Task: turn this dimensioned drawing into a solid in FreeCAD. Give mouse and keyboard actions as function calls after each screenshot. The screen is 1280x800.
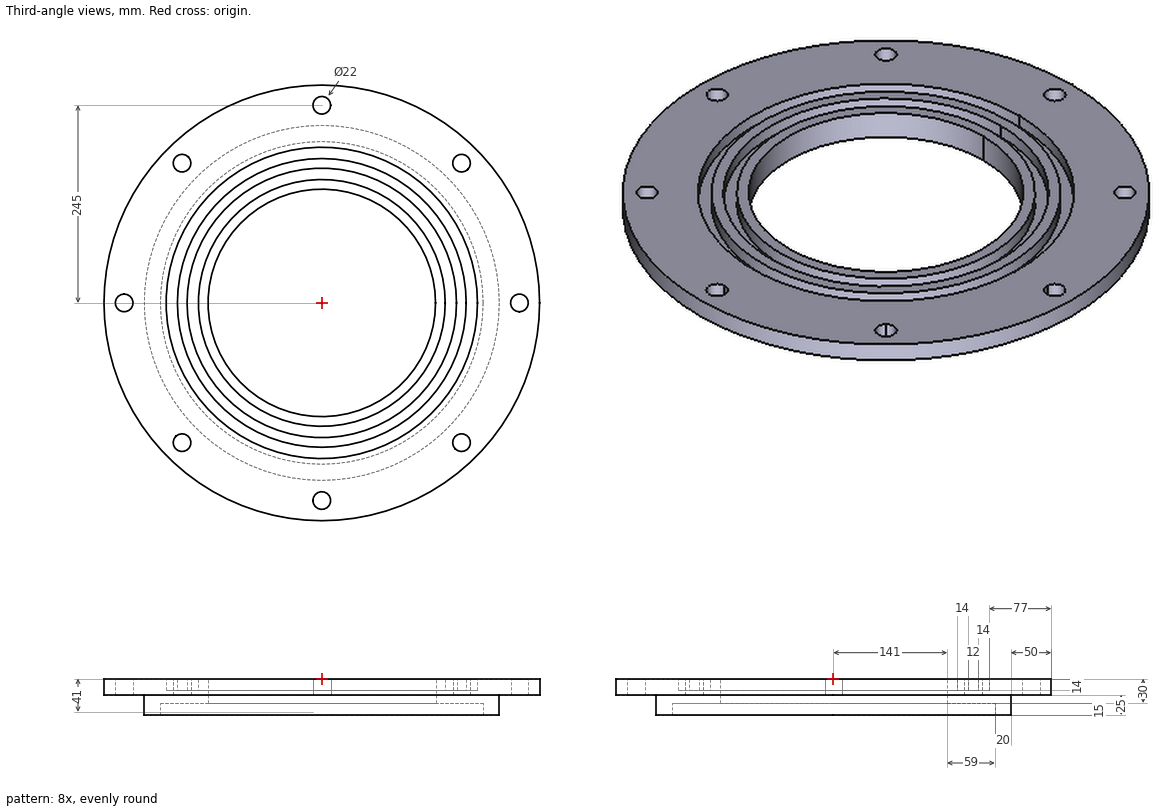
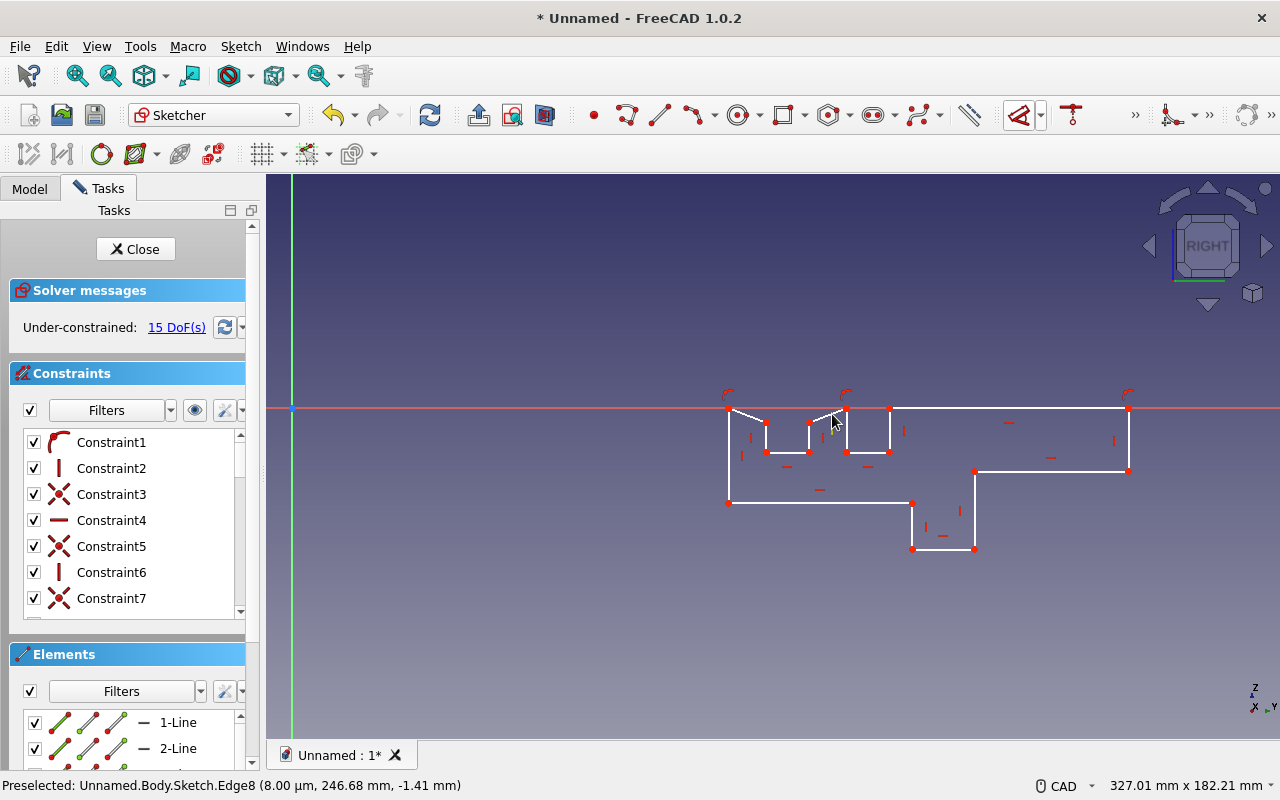
click(832, 414)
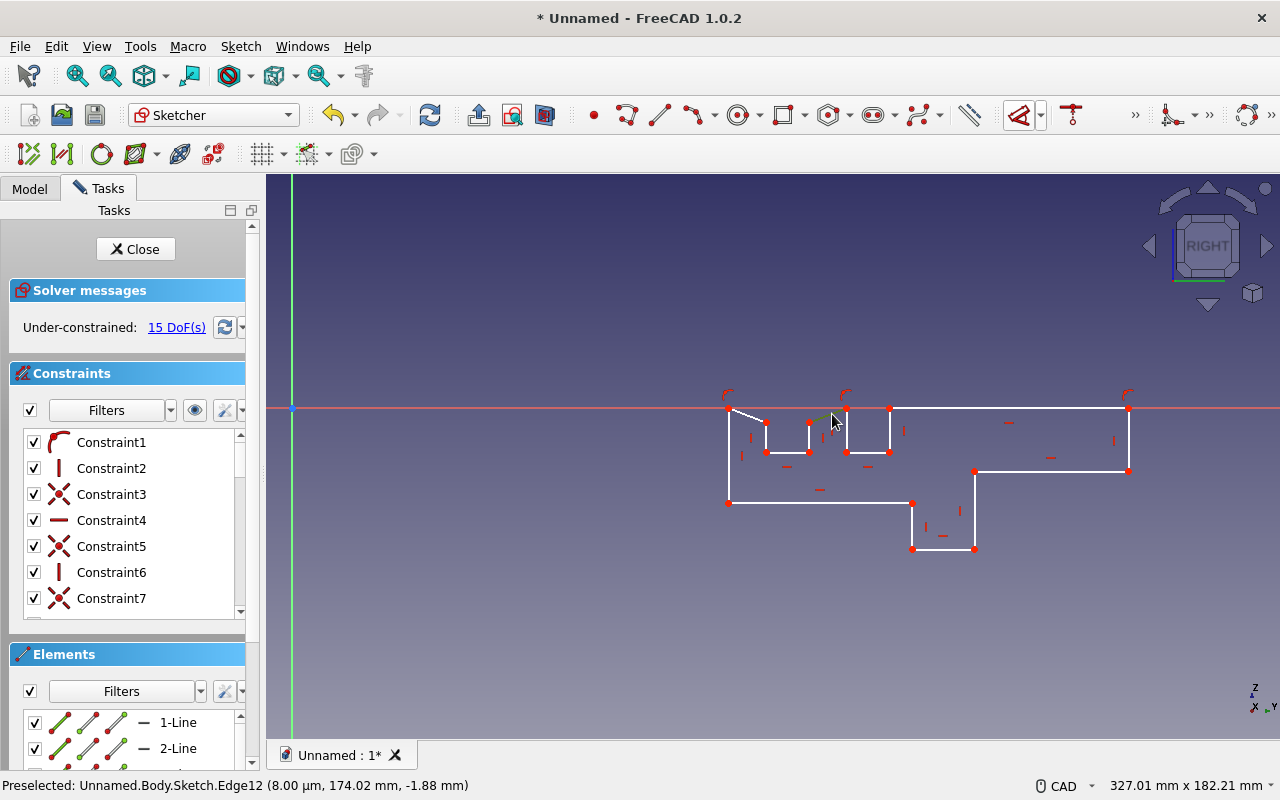
key(h)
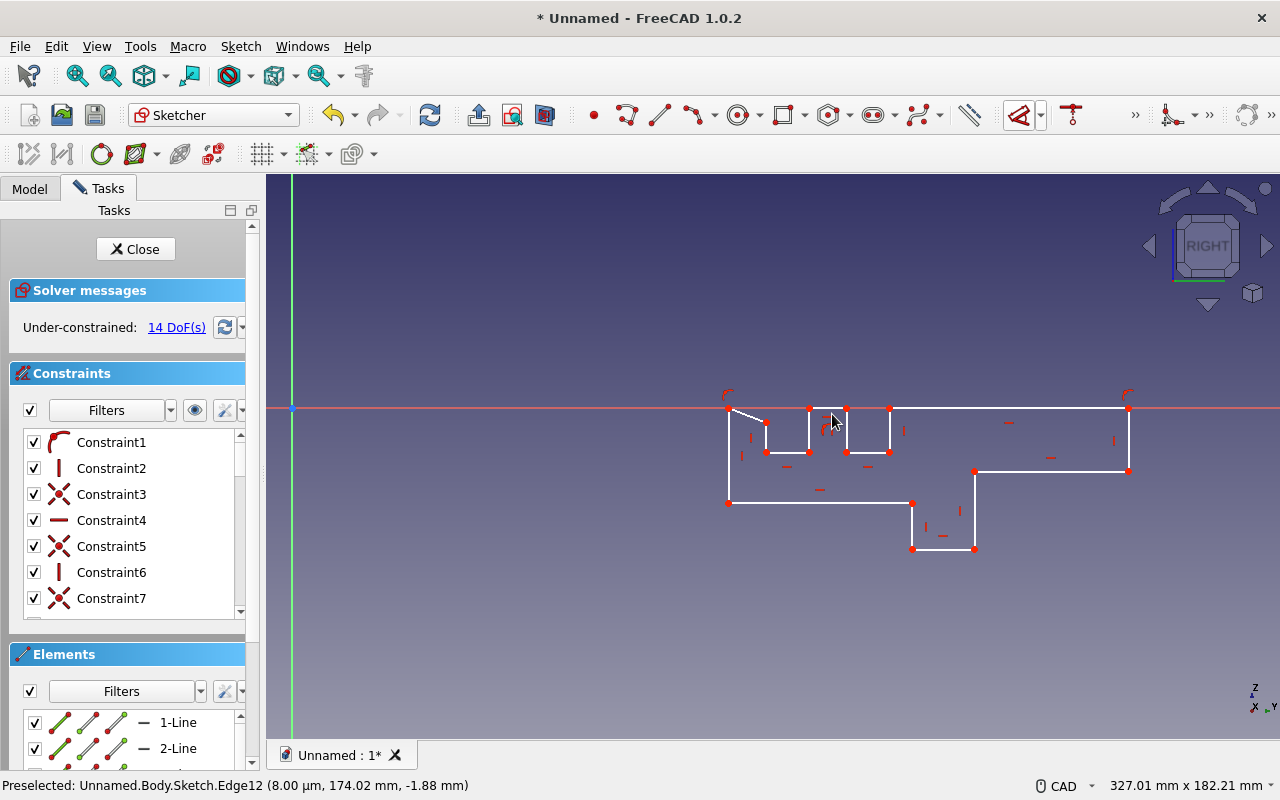
scroll(755, 418, up, 2)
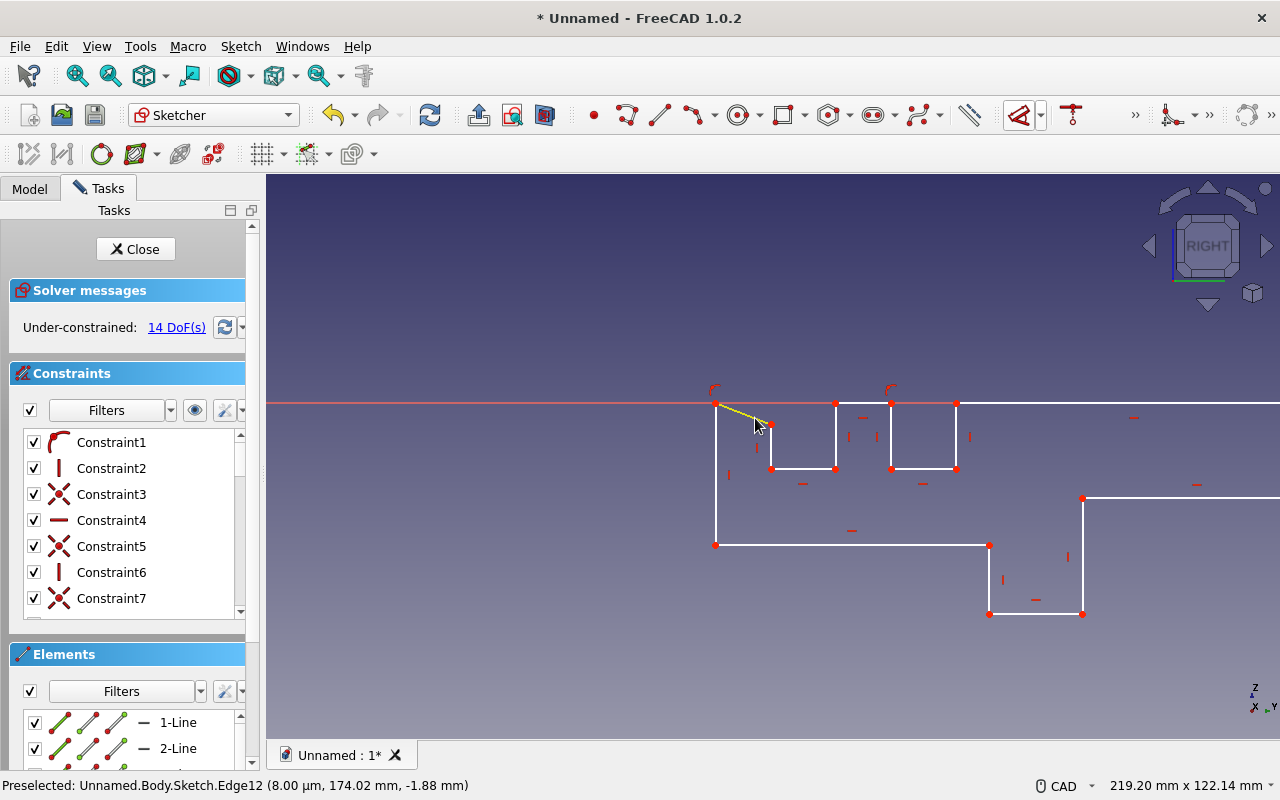
click(755, 418)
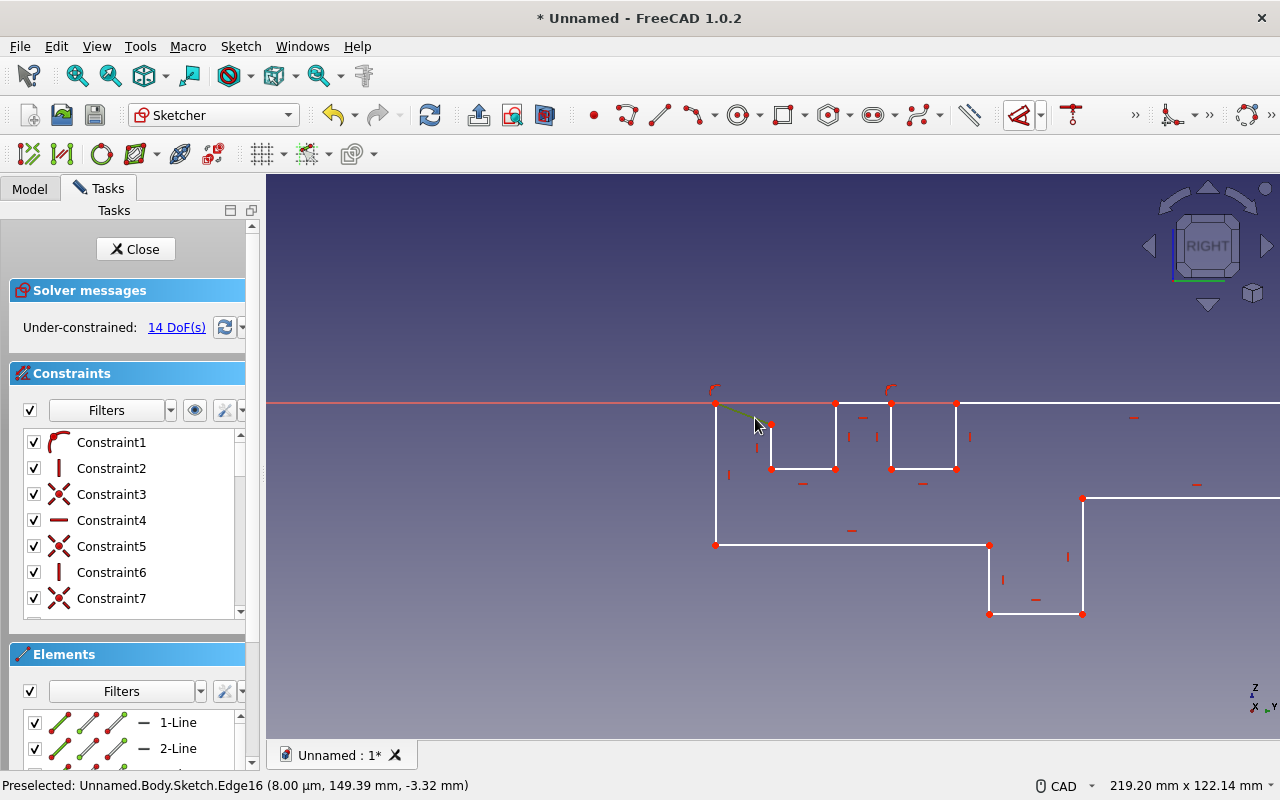
key(h)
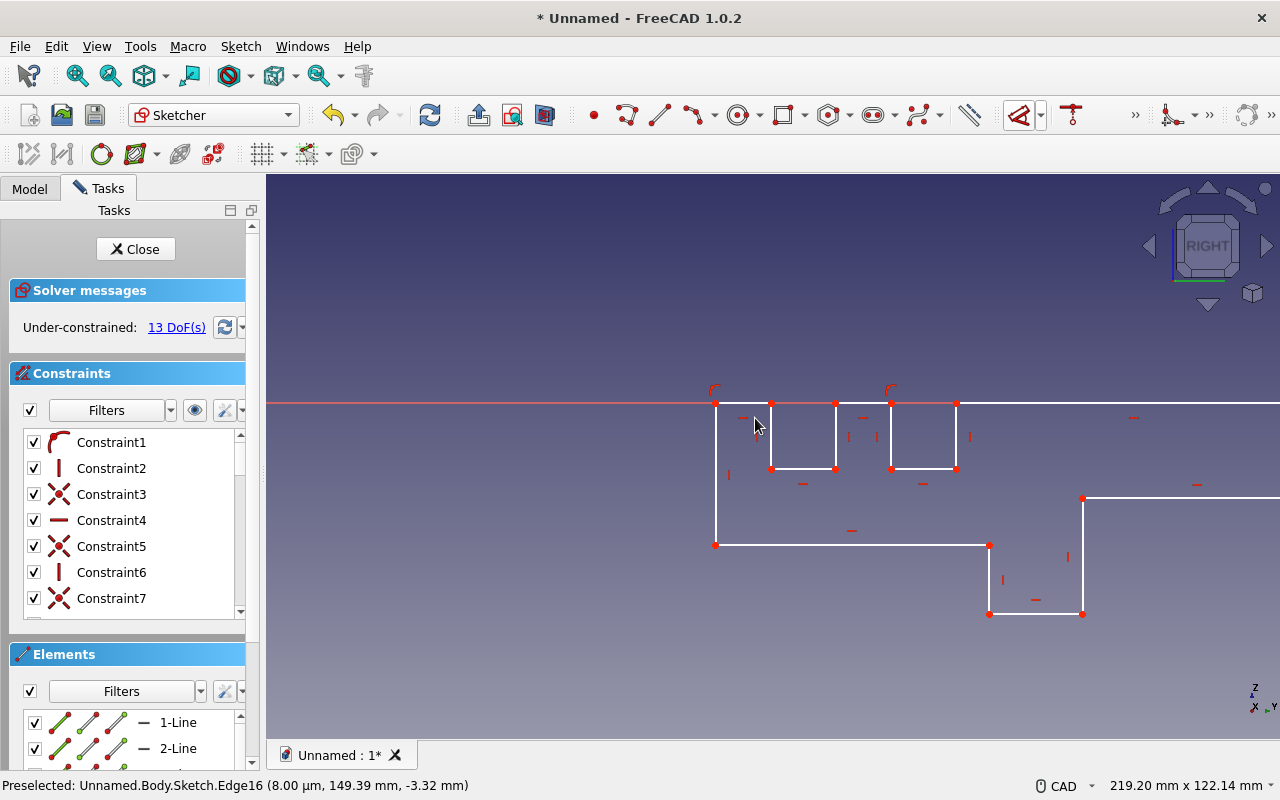
click(716, 446)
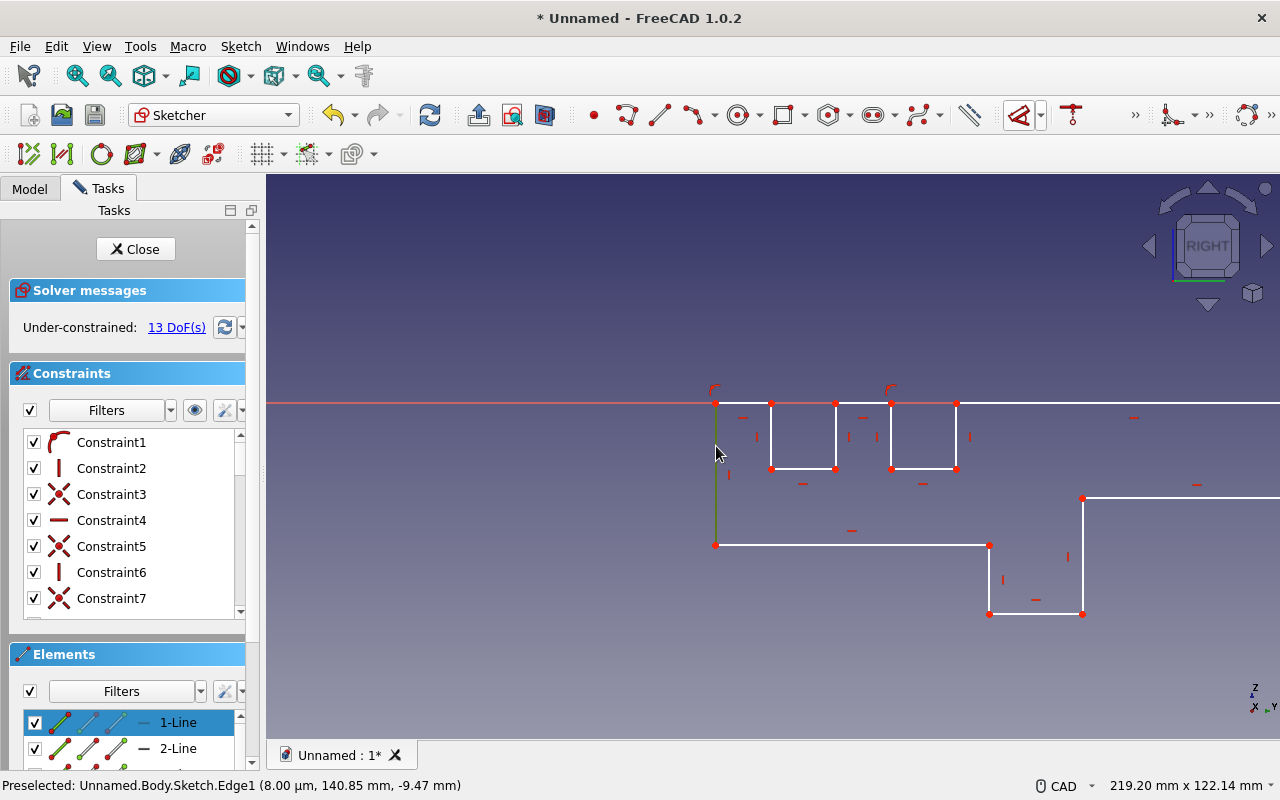
key(i)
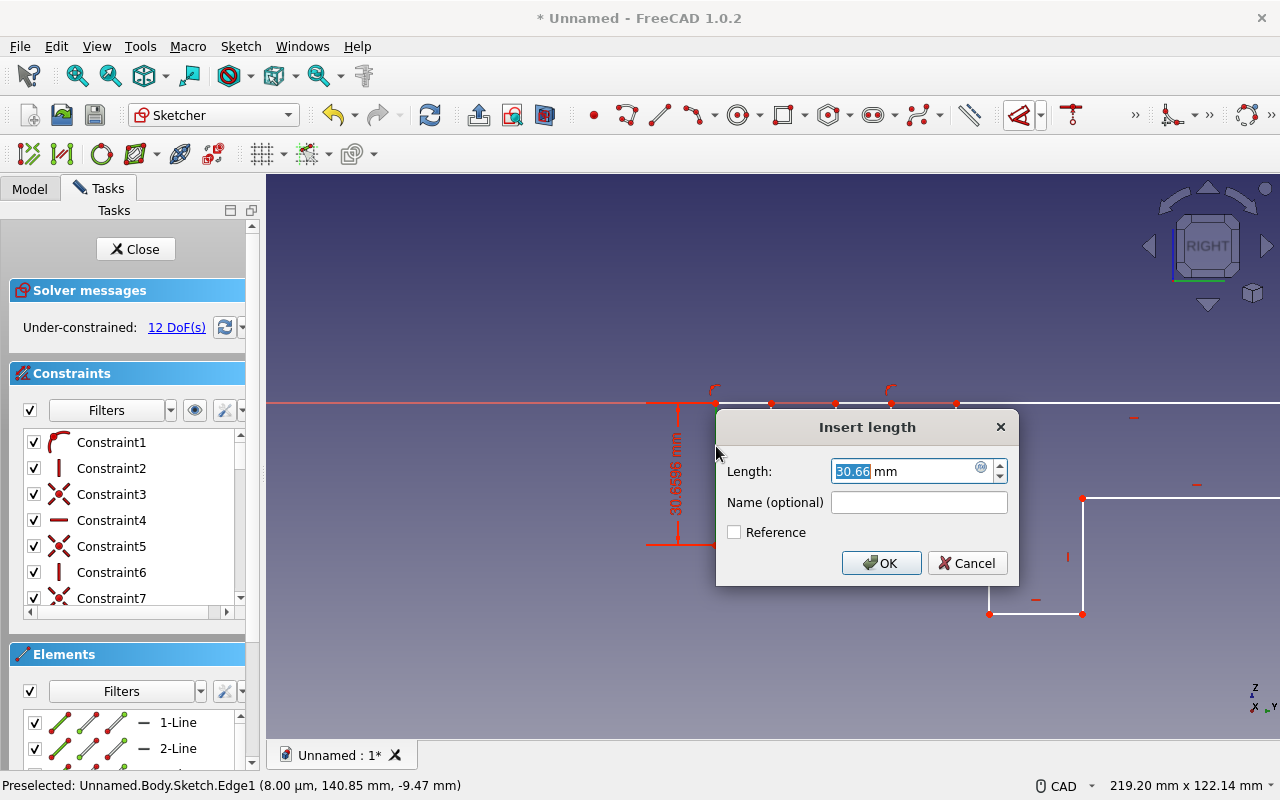
text(30)
key(Return)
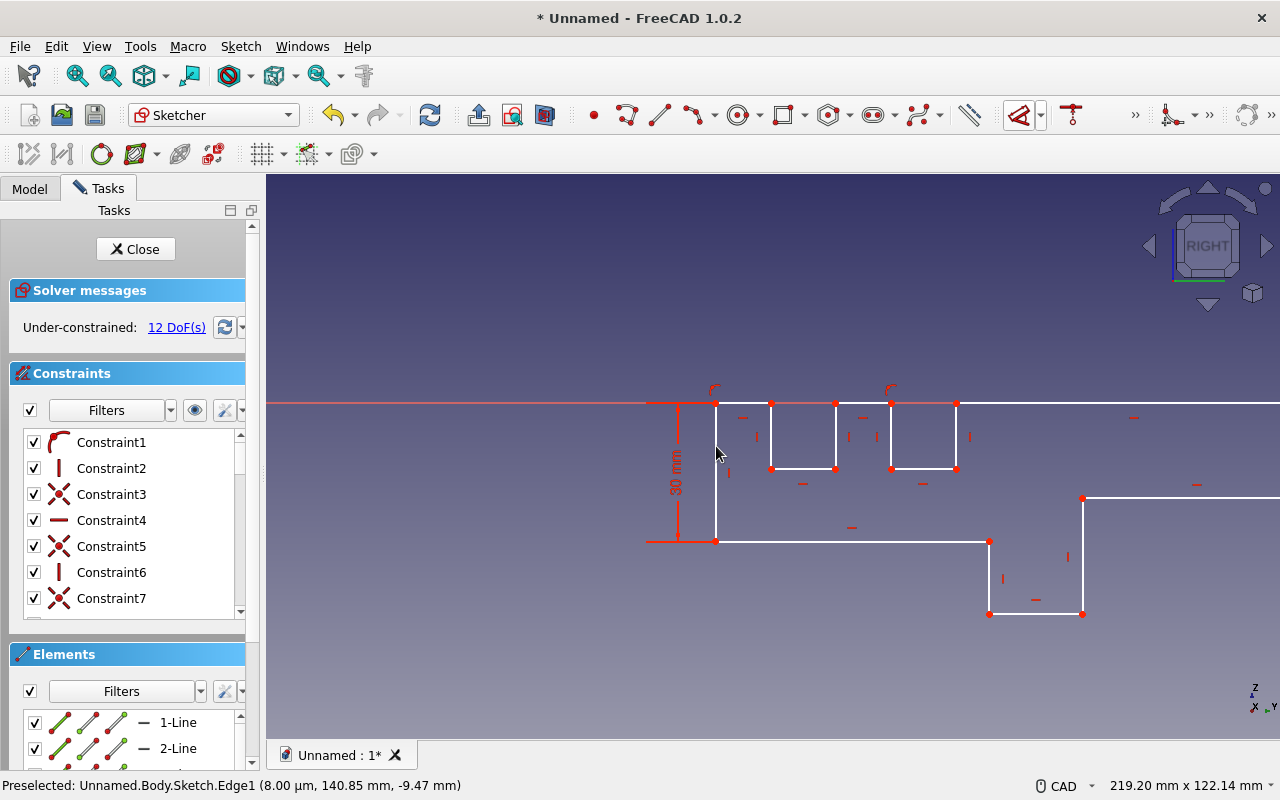
click(798, 542)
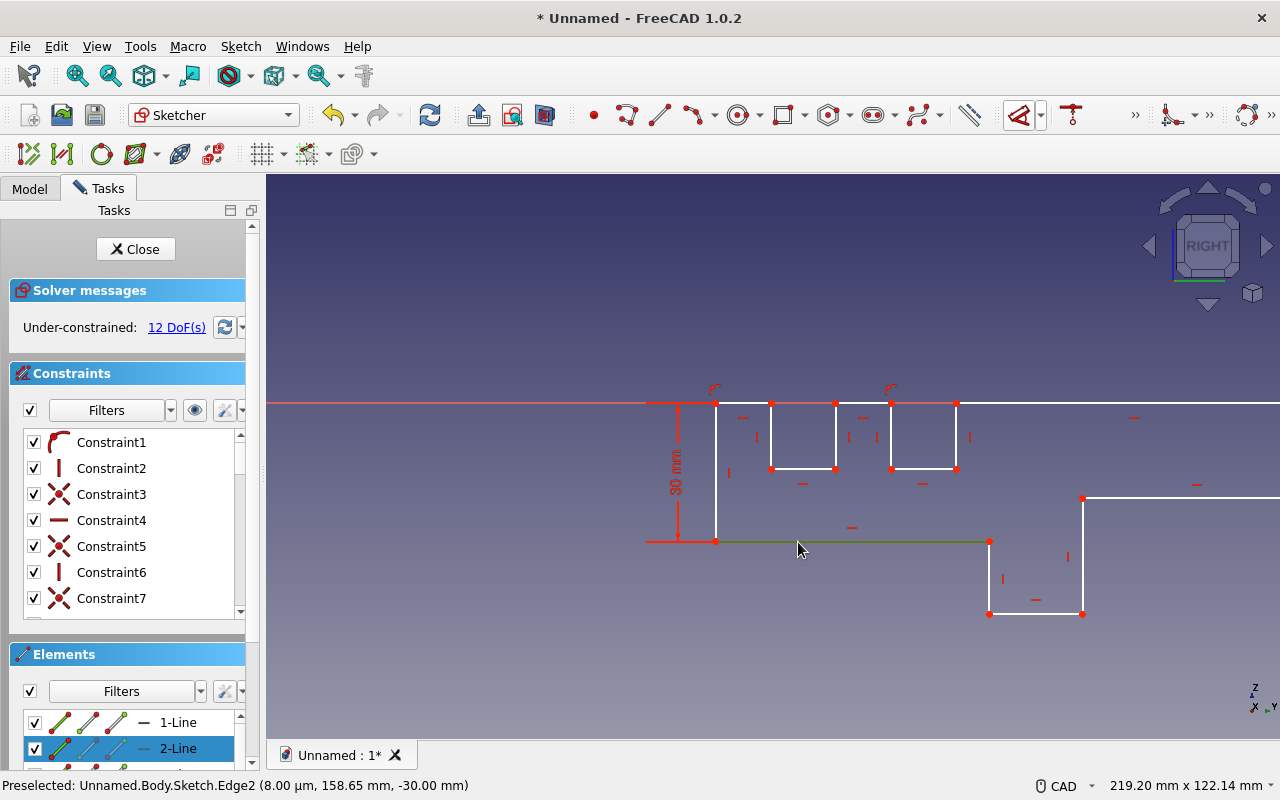
click(1040, 116)